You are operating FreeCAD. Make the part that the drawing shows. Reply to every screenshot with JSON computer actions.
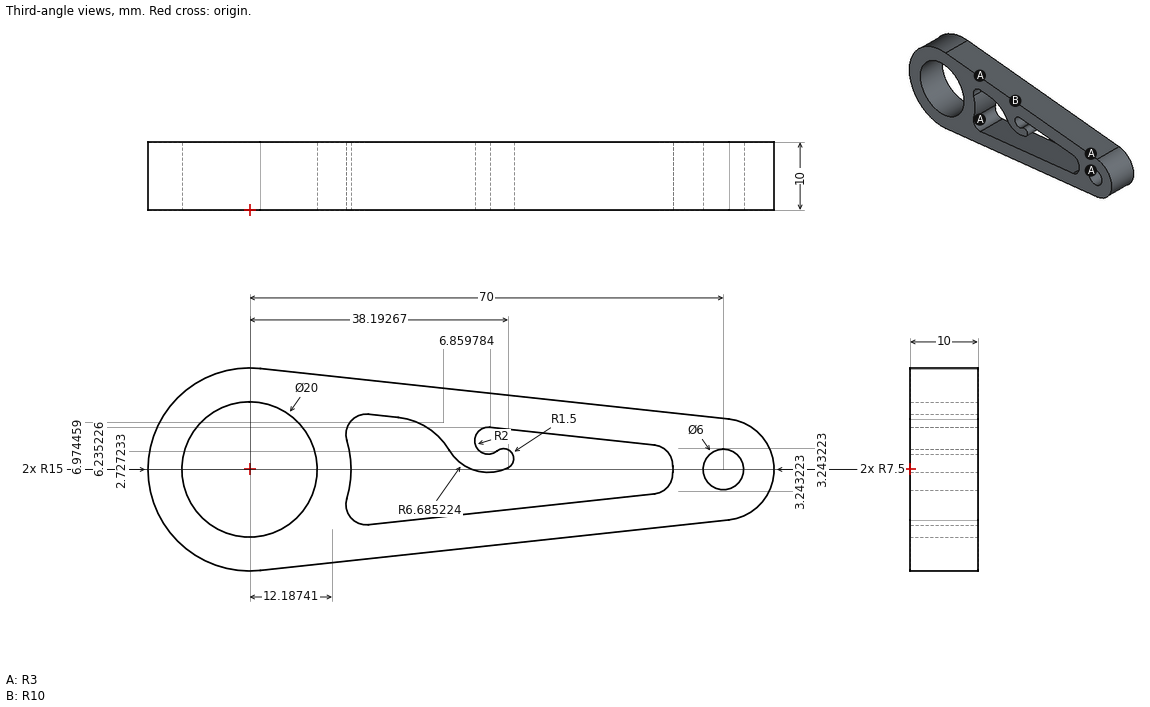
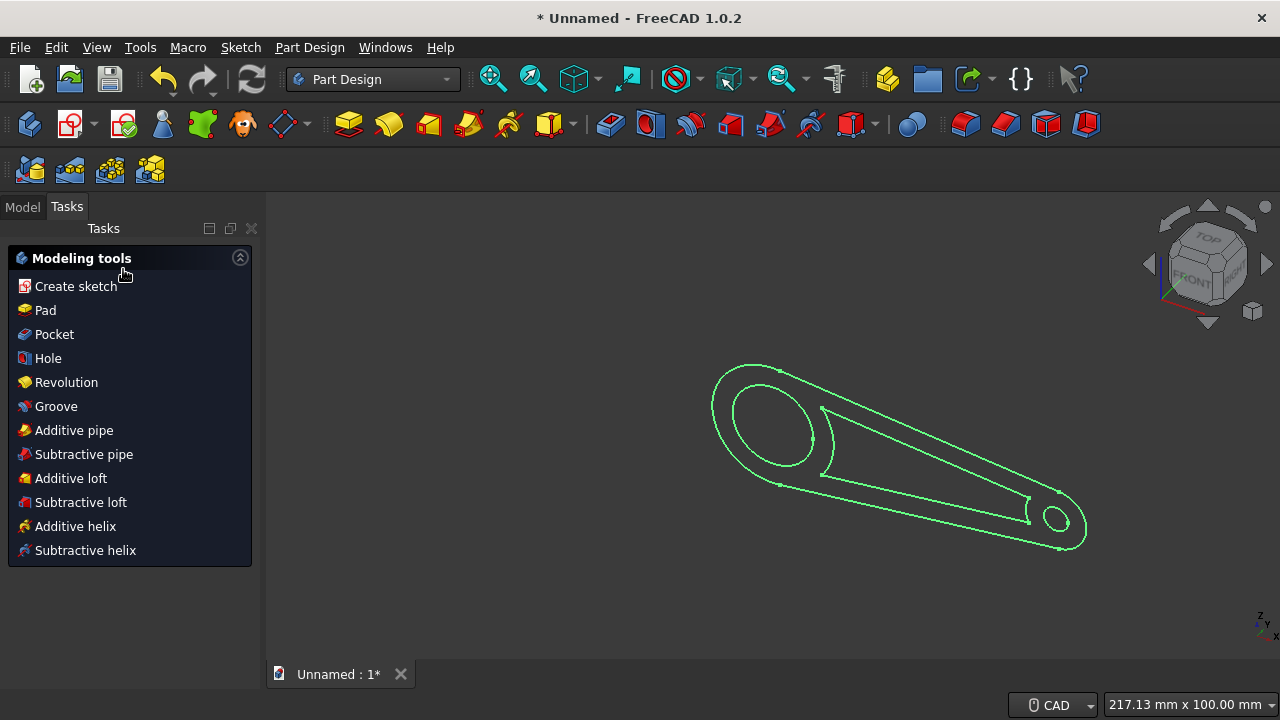
{"action": "left_click", "coordinate": [350, 124]}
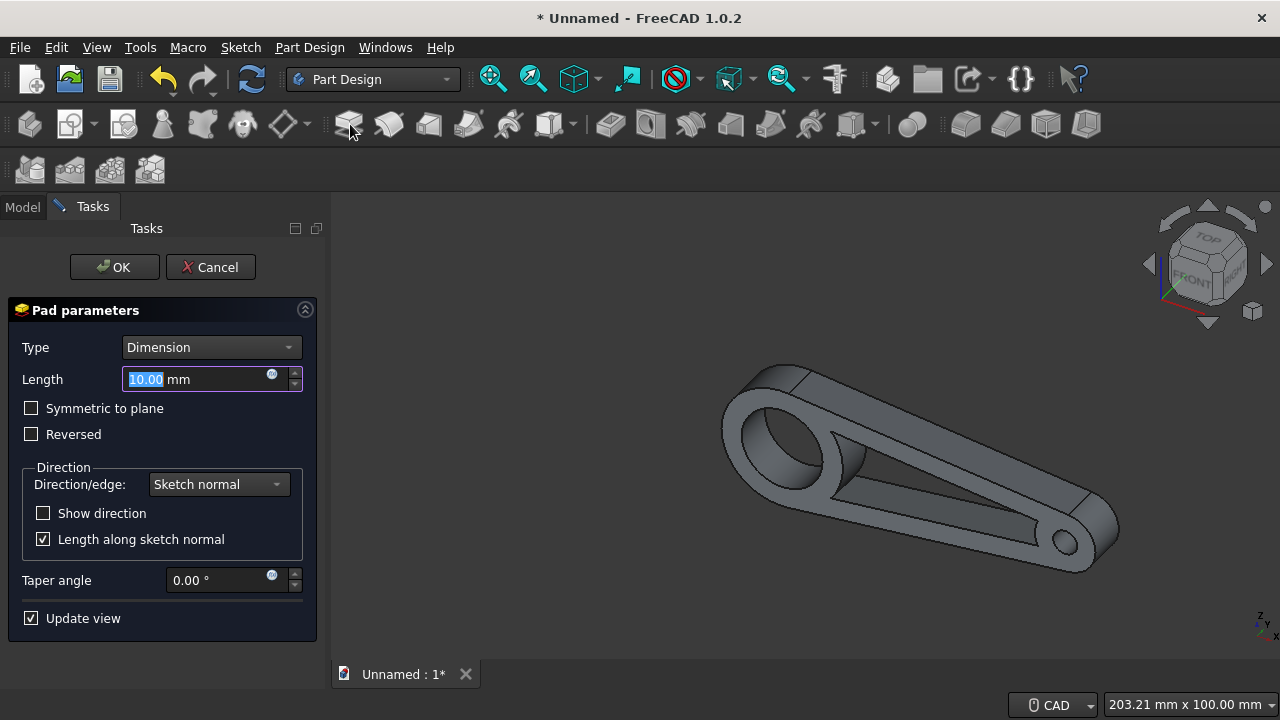
{"action": "type", "text": "10"}
{"action": "key", "text": "Tab"}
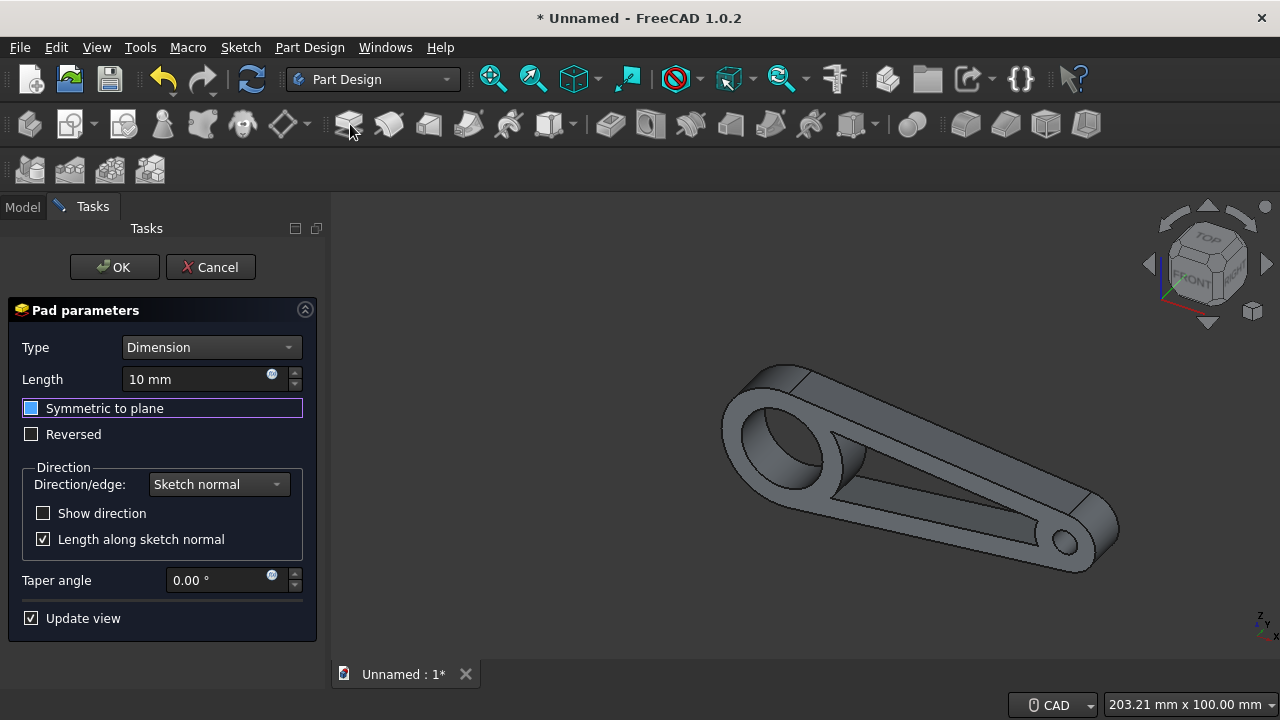
{"action": "left_click", "coordinate": [30, 434]}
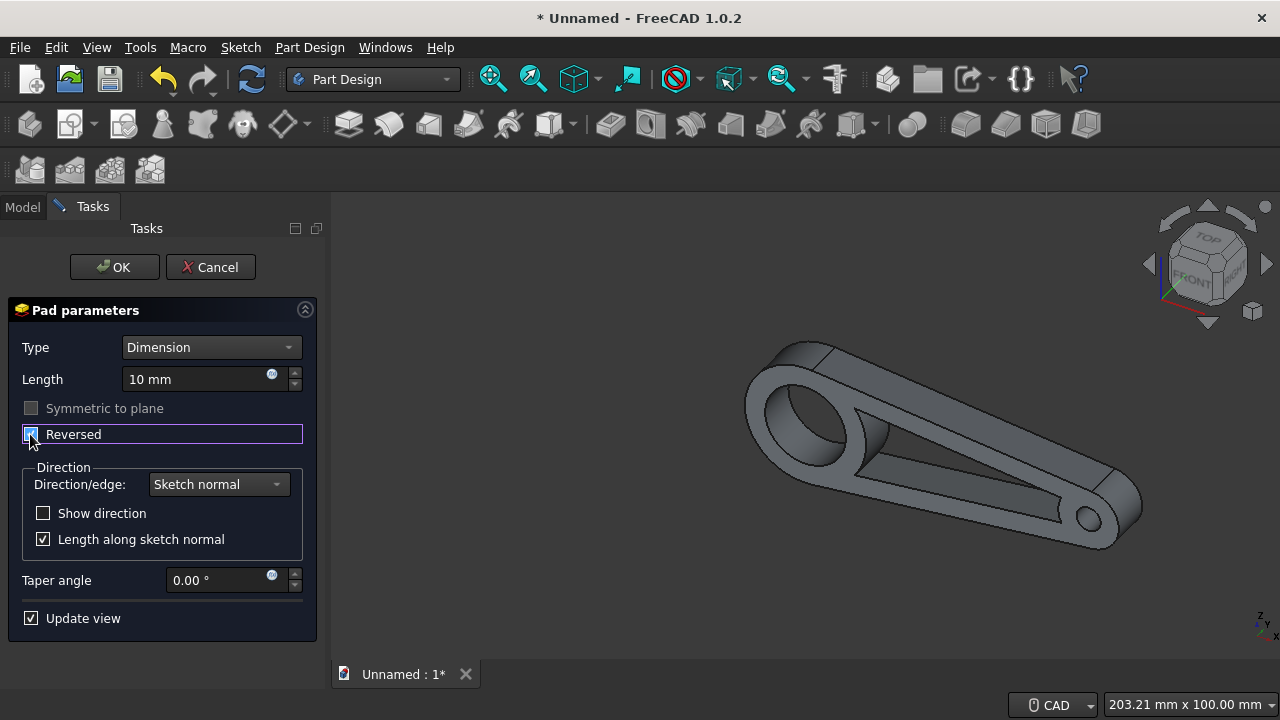
{"action": "left_click", "coordinate": [115, 267]}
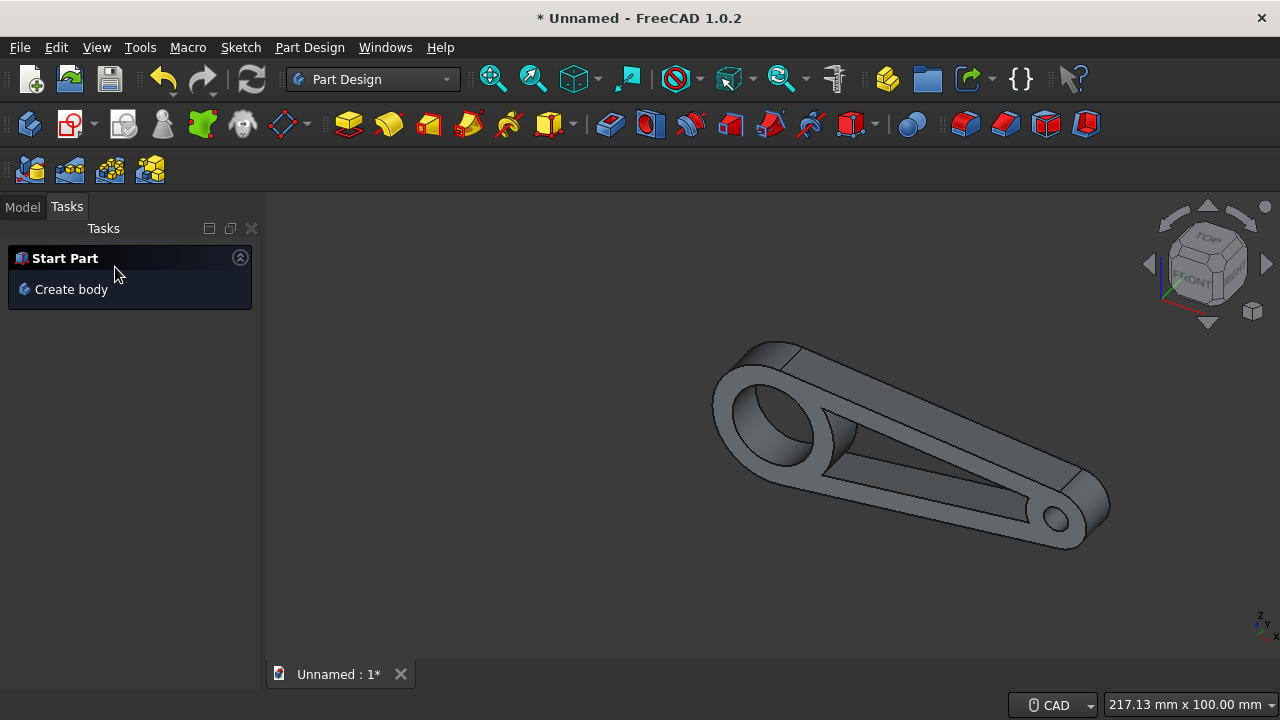
{"action": "key", "text": "0"}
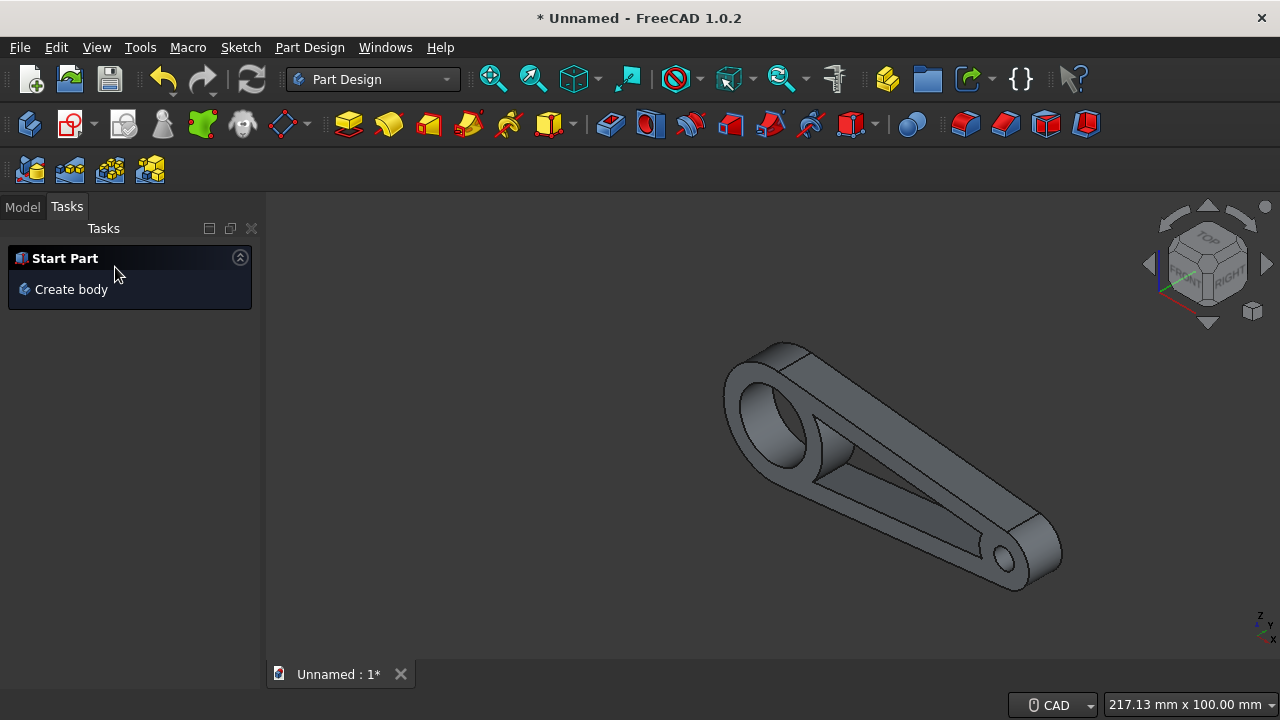
{"action": "key", "text": "2"}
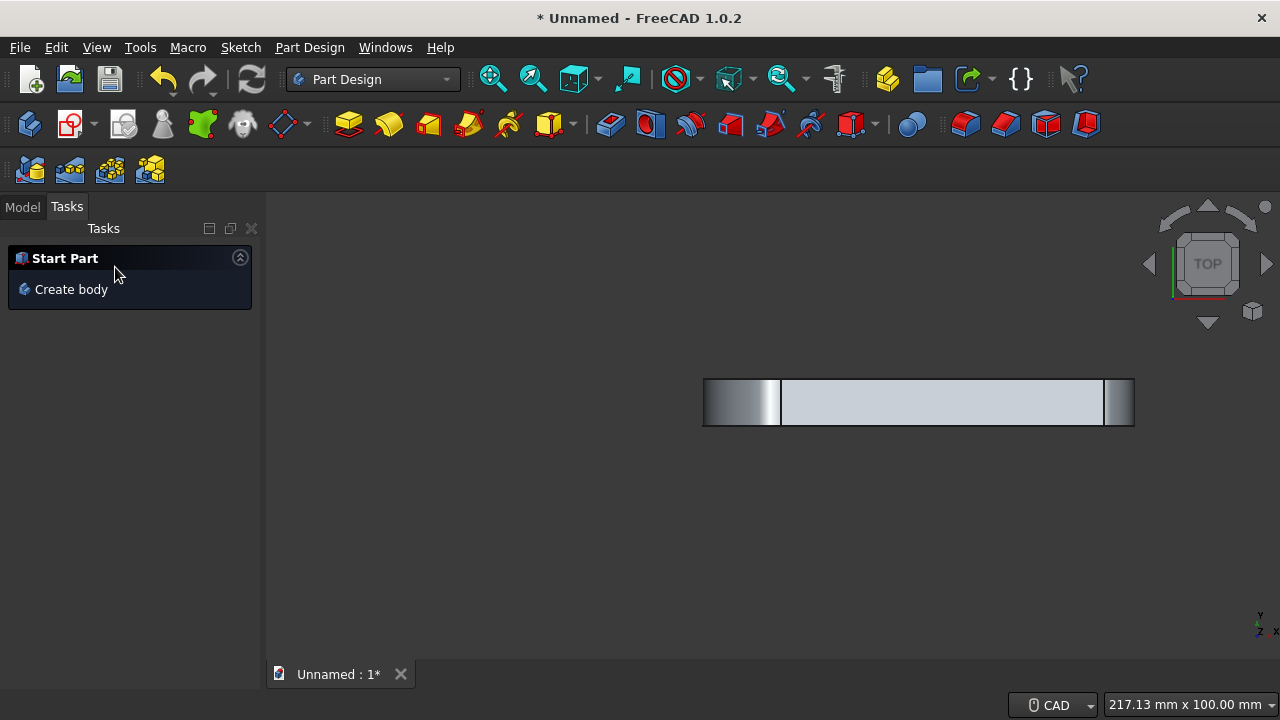
{"action": "left_click", "coordinate": [494, 80]}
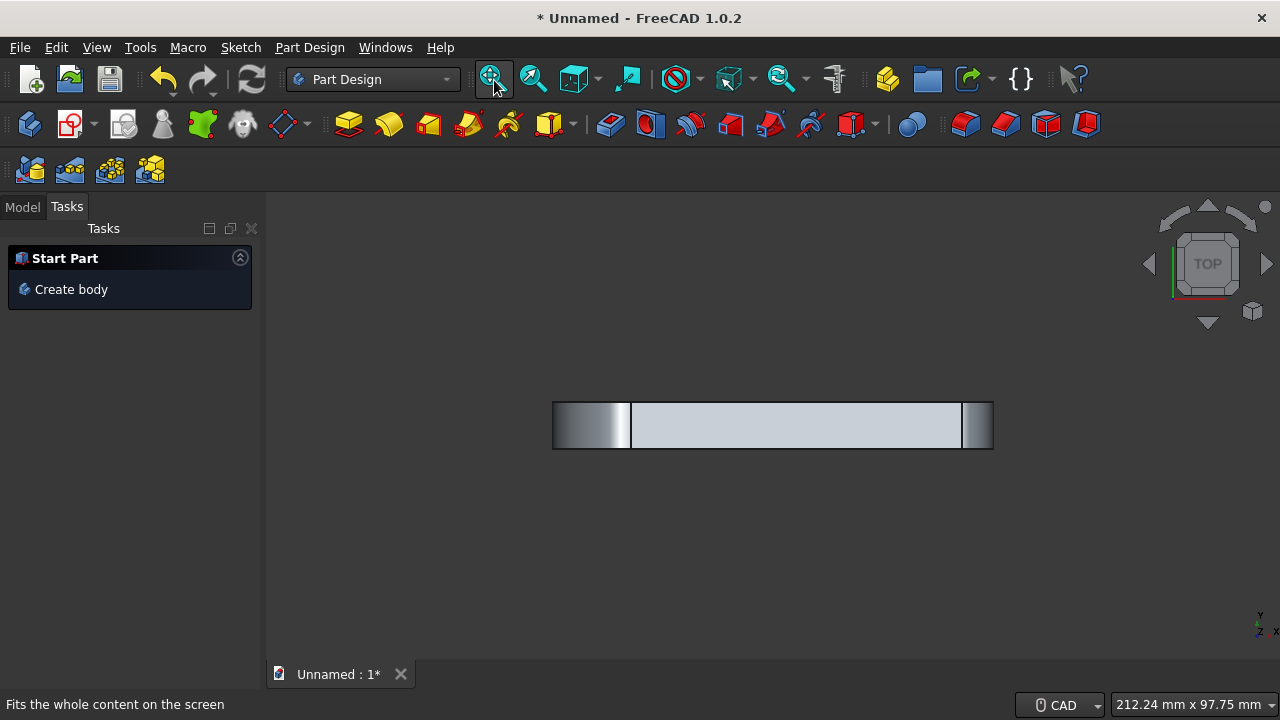
{"action": "key", "text": "1"}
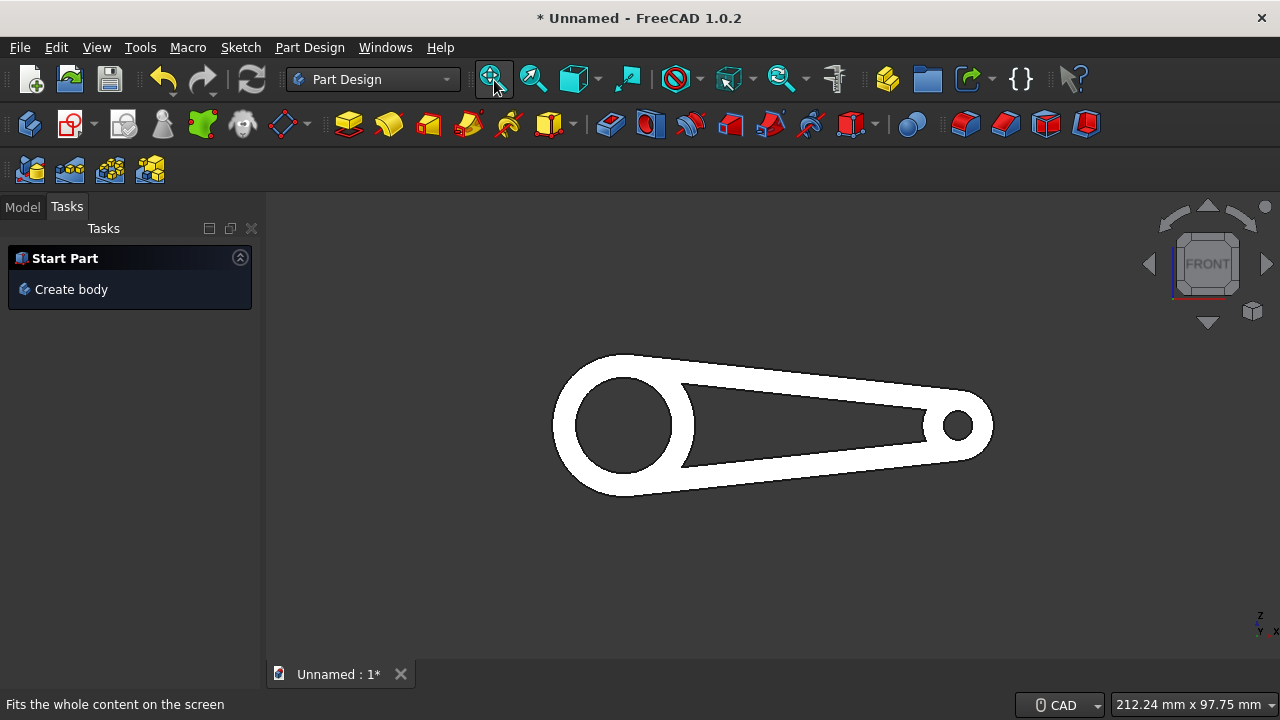
{"action": "left_click", "coordinate": [494, 80]}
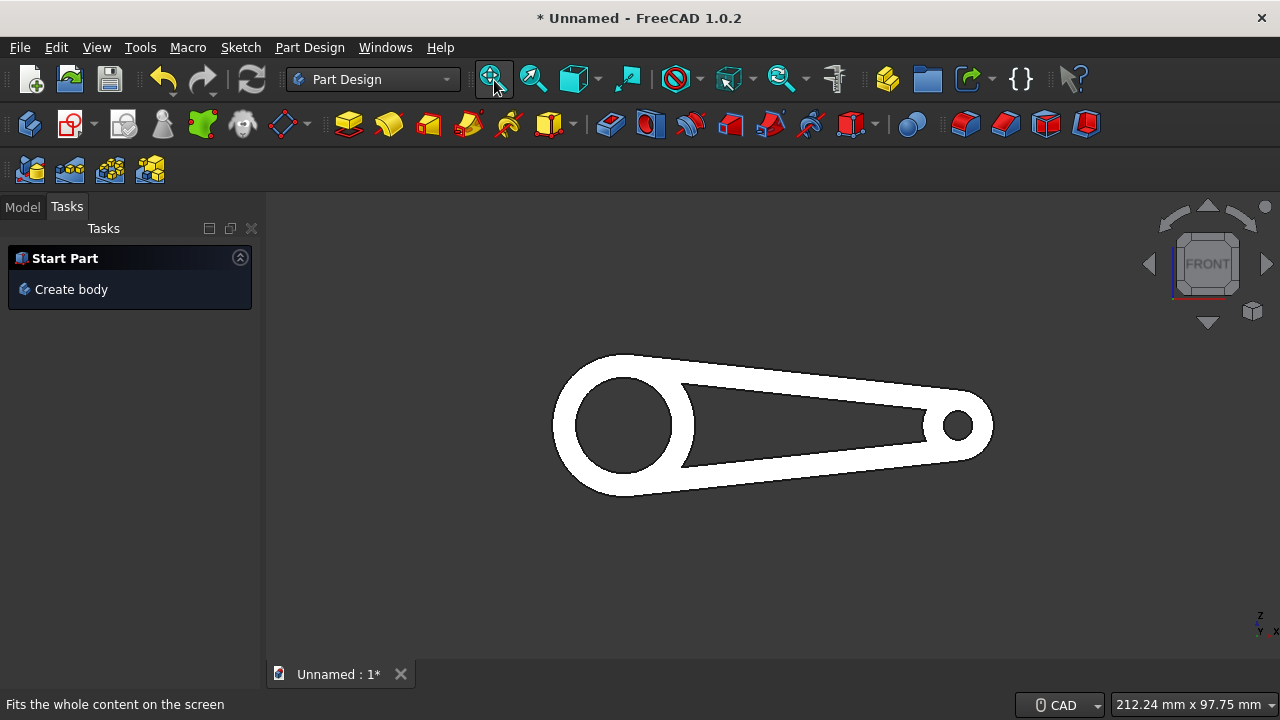
{"action": "key", "text": "3"}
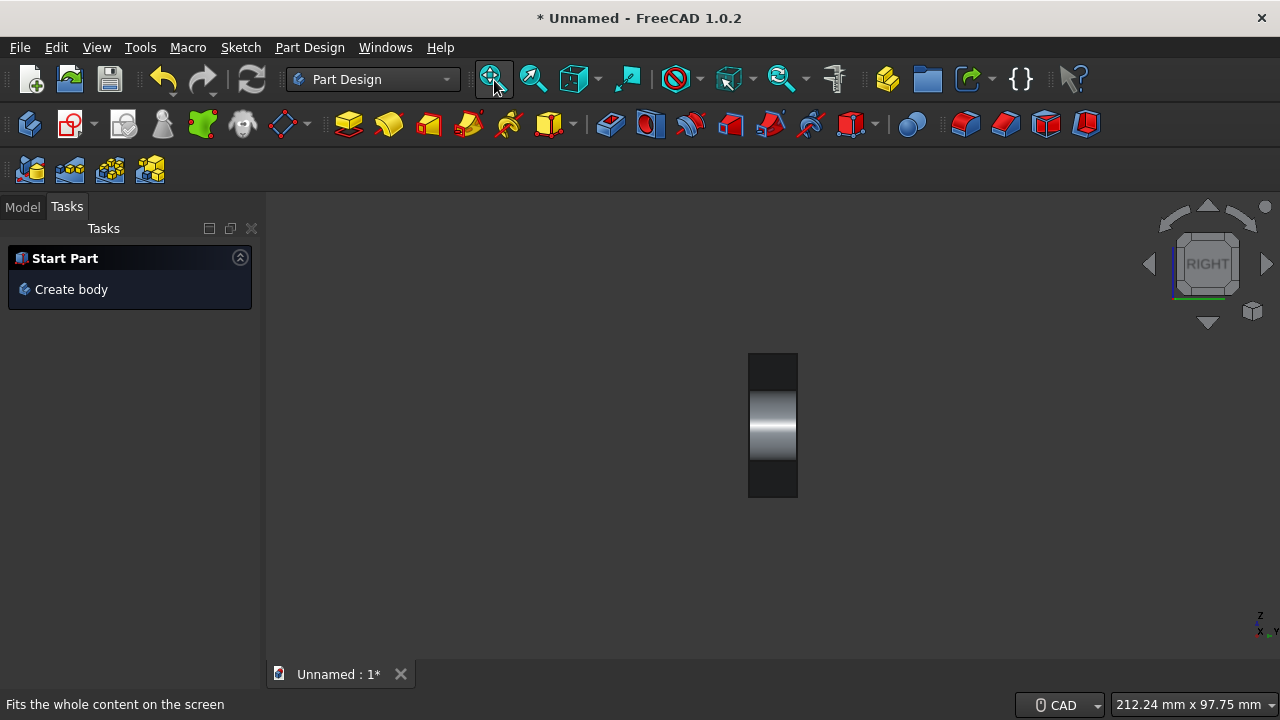
{"action": "left_click", "coordinate": [494, 80]}